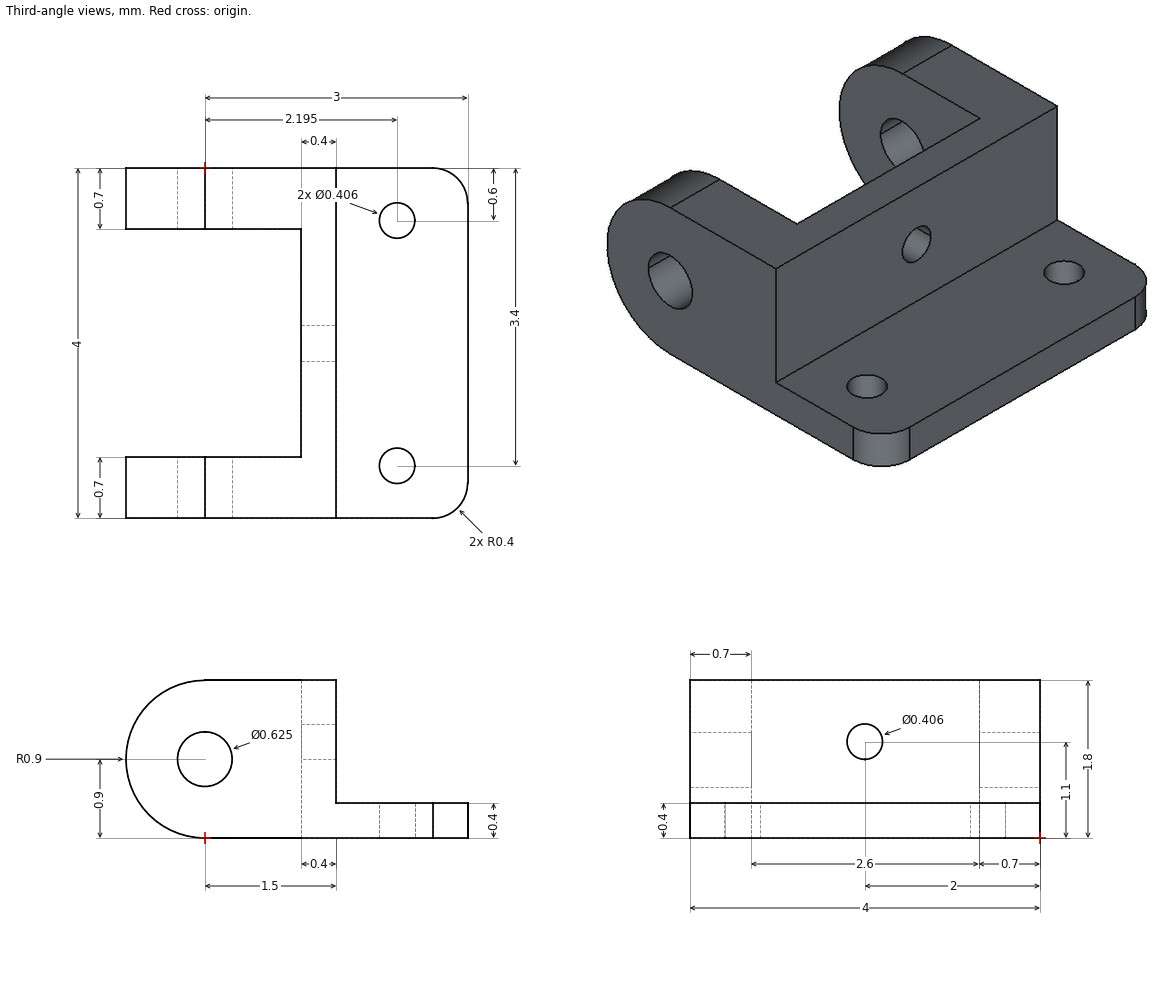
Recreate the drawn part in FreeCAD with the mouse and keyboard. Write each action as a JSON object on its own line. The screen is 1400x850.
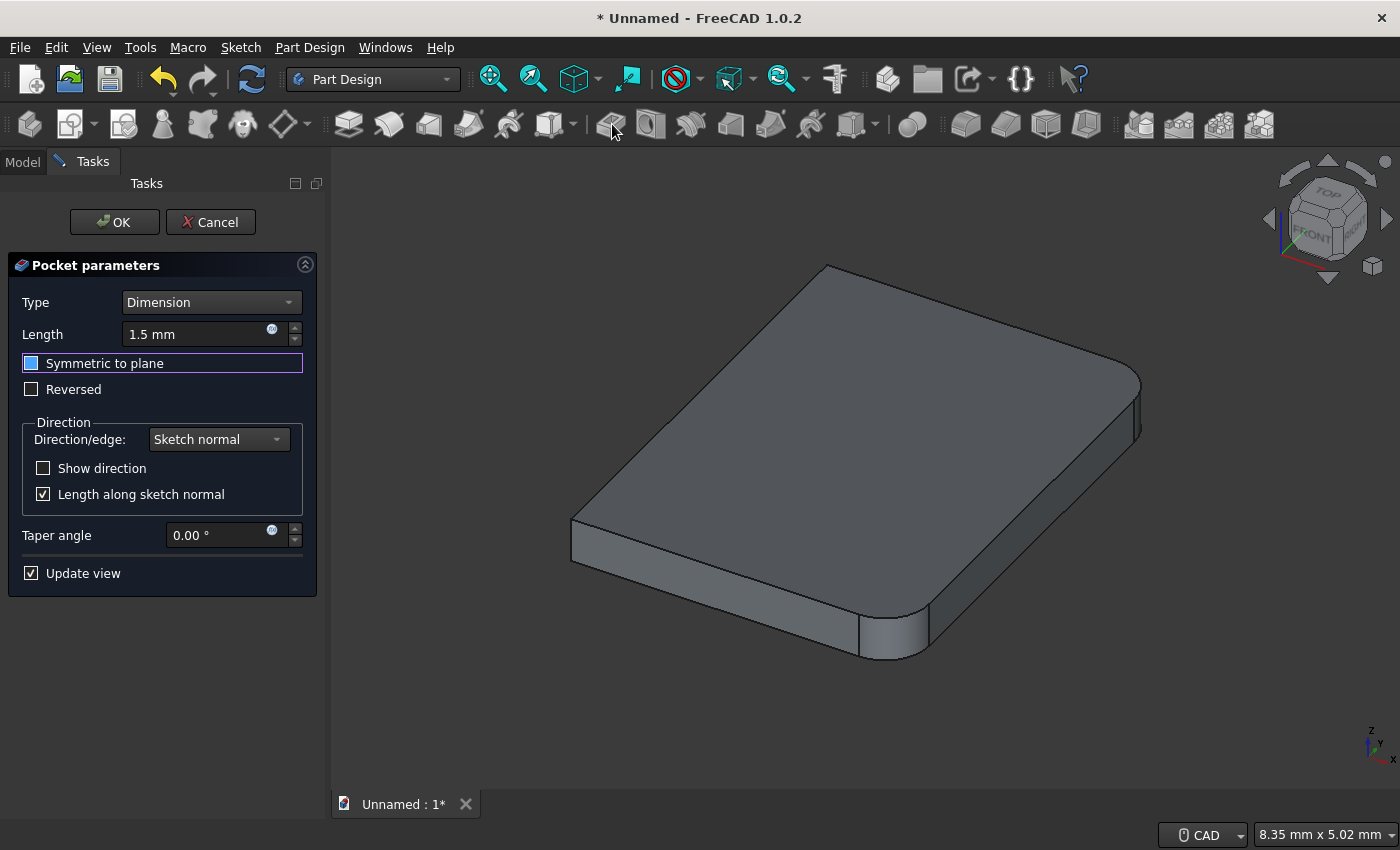
{"action": "left_click", "coordinate": [30, 389]}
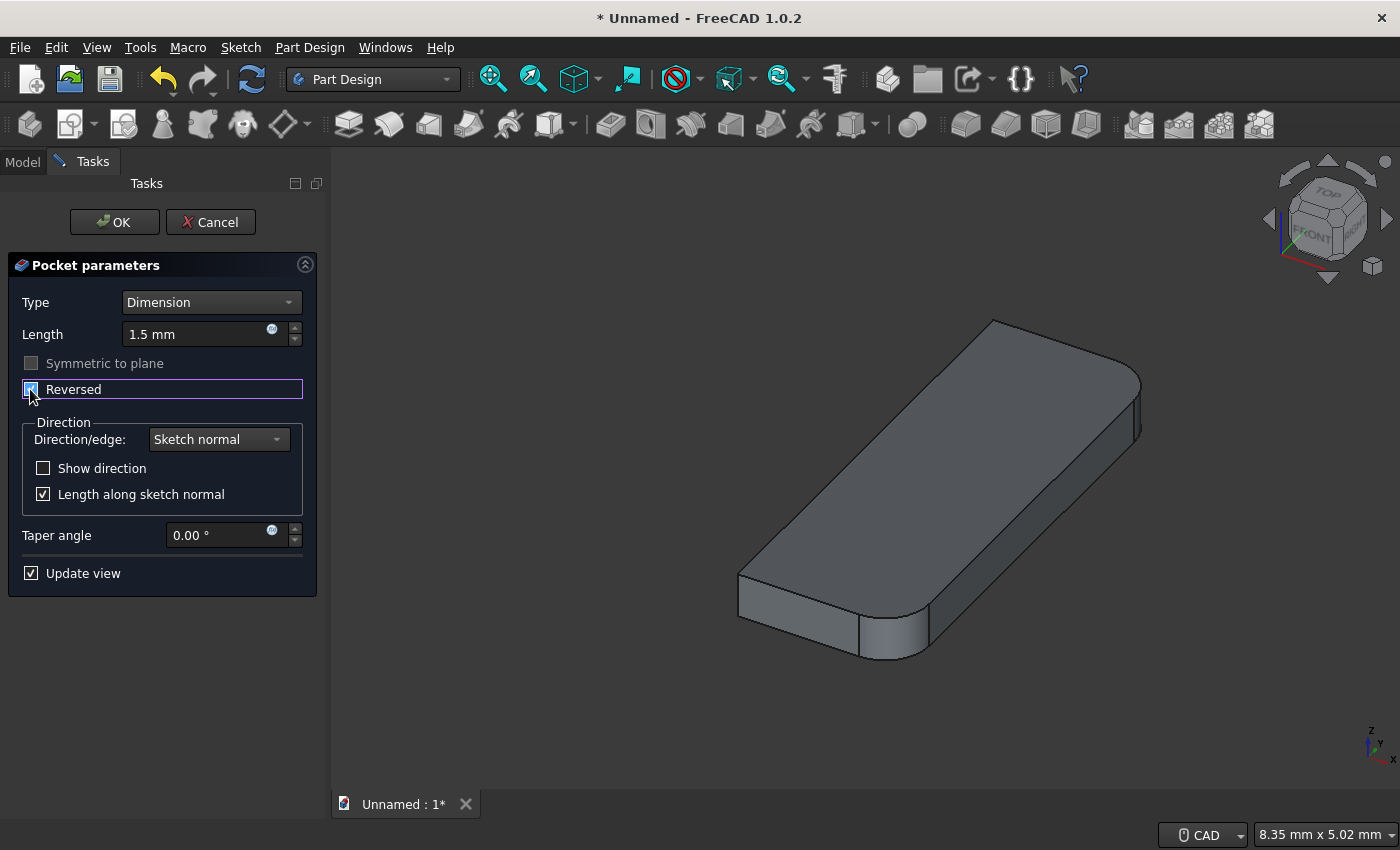
{"action": "left_click", "coordinate": [115, 222]}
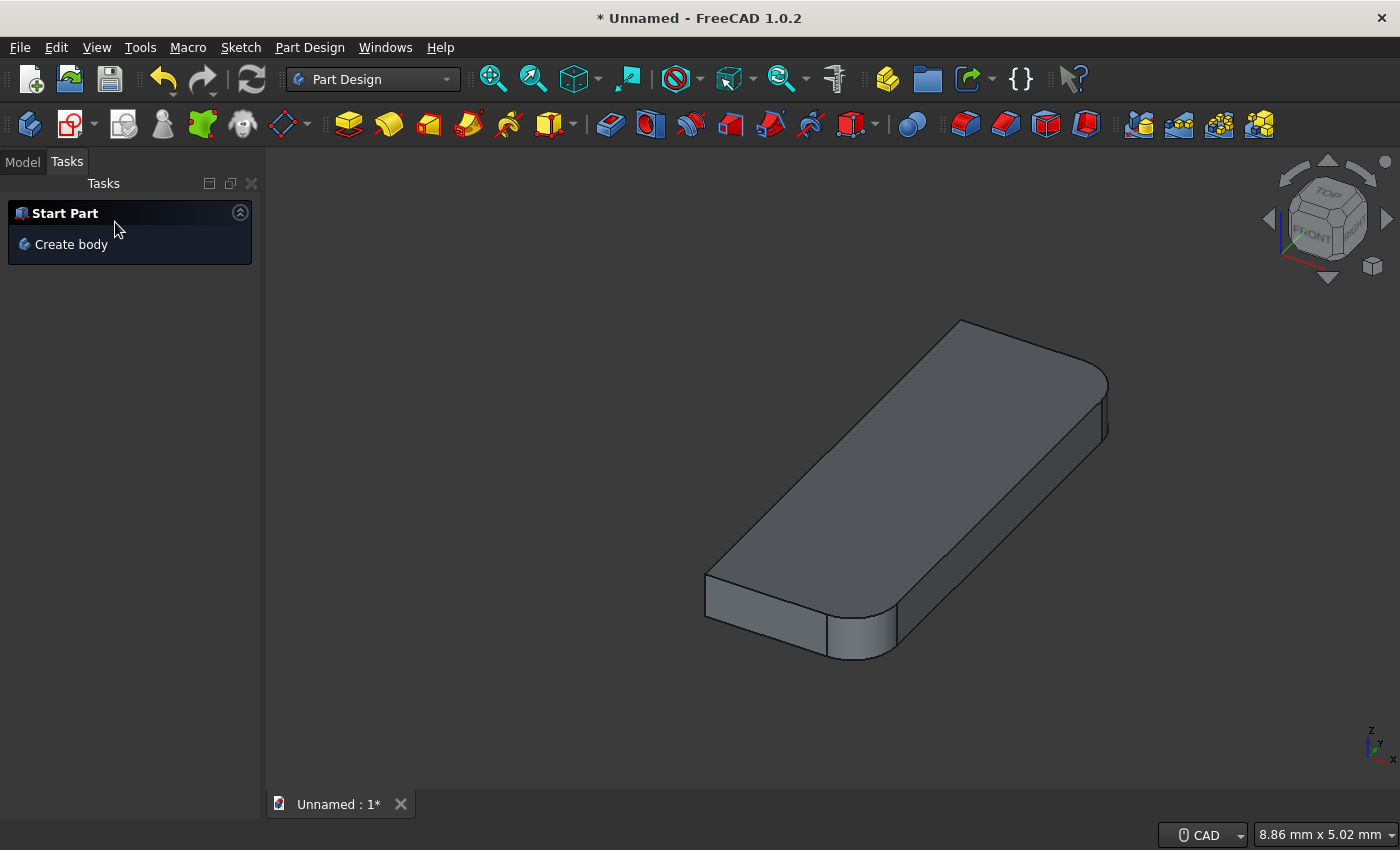
{"action": "left_click", "coordinate": [70, 124]}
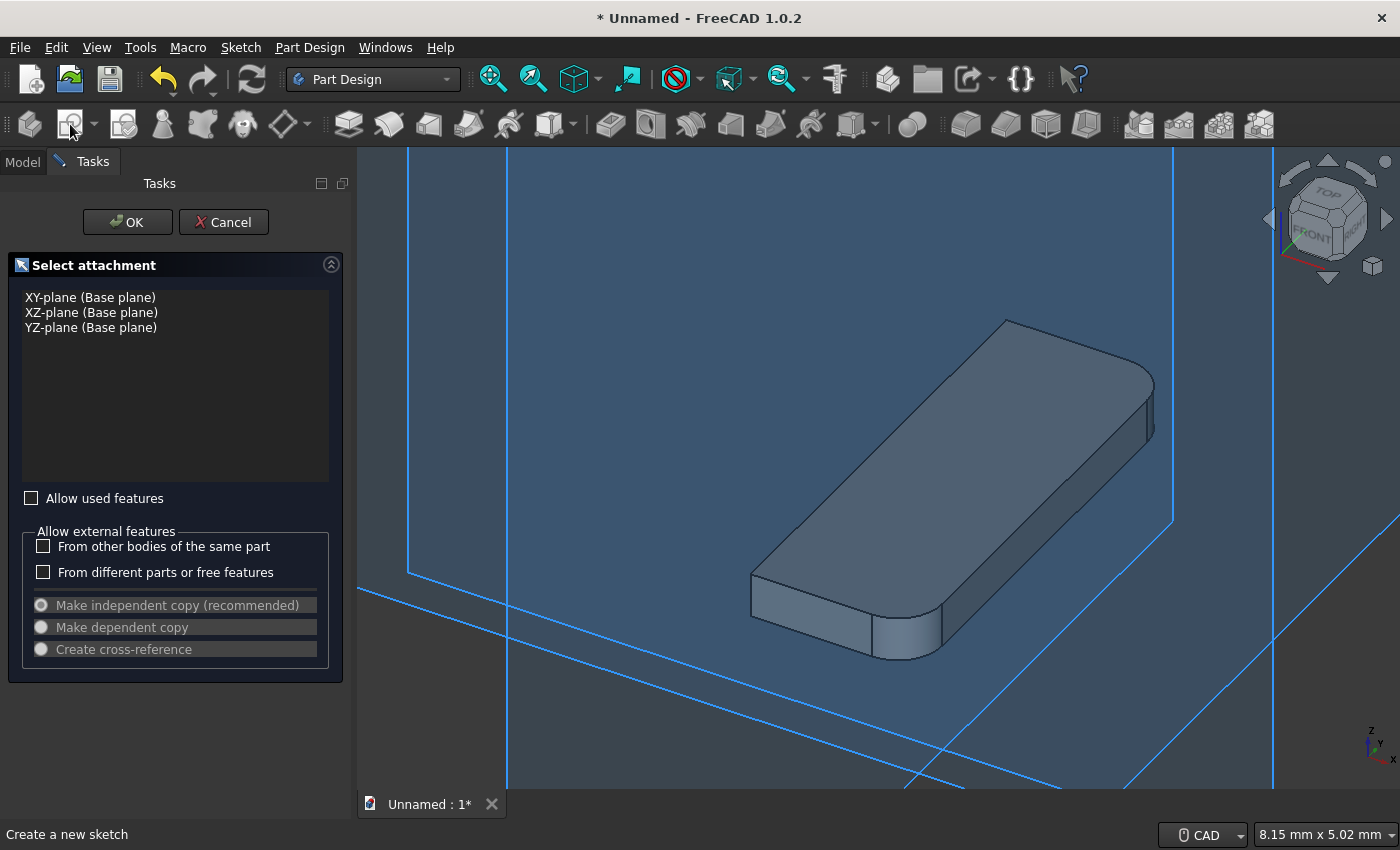
{"action": "left_click", "coordinate": [82, 312]}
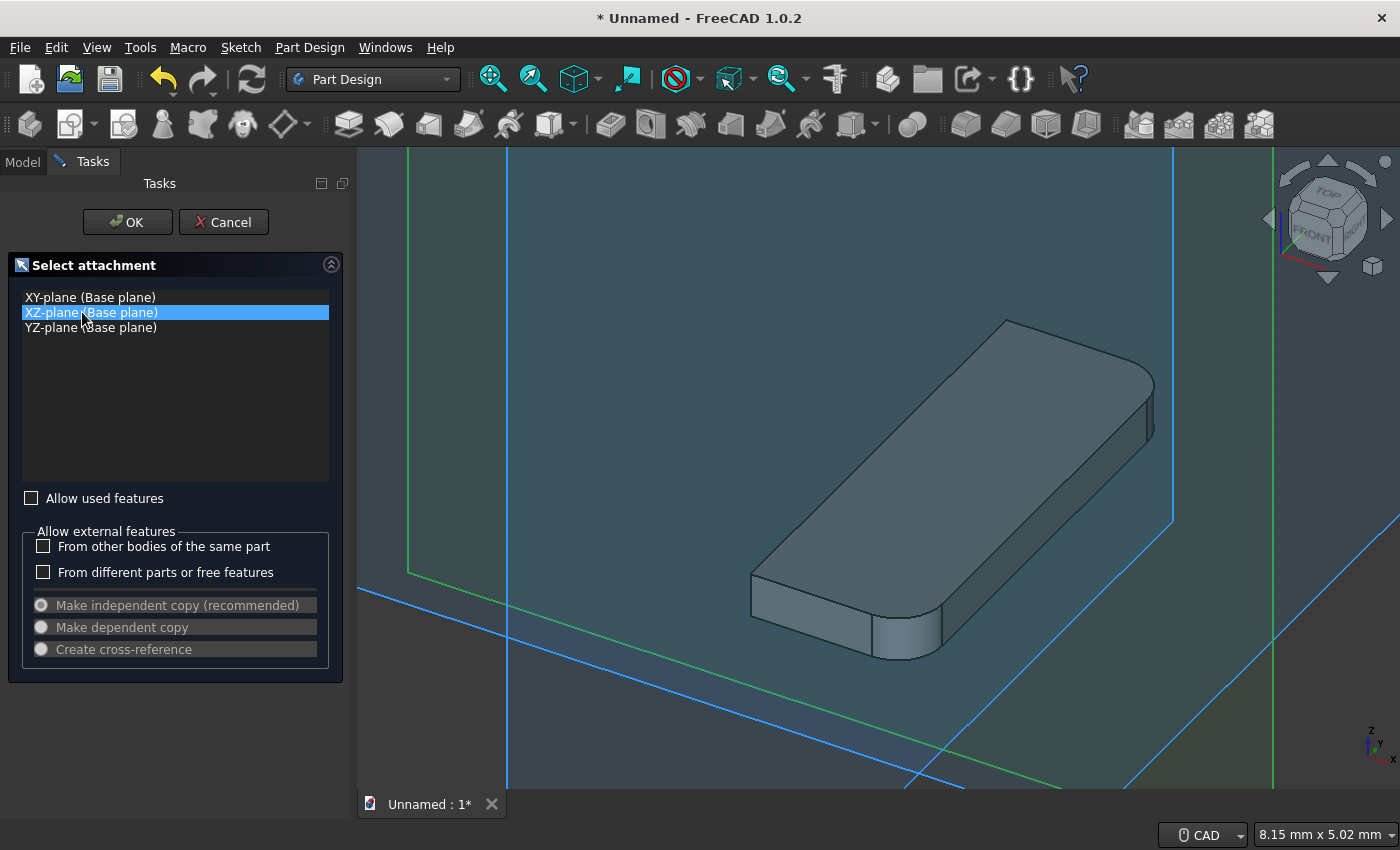
{"action": "left_click", "coordinate": [128, 222]}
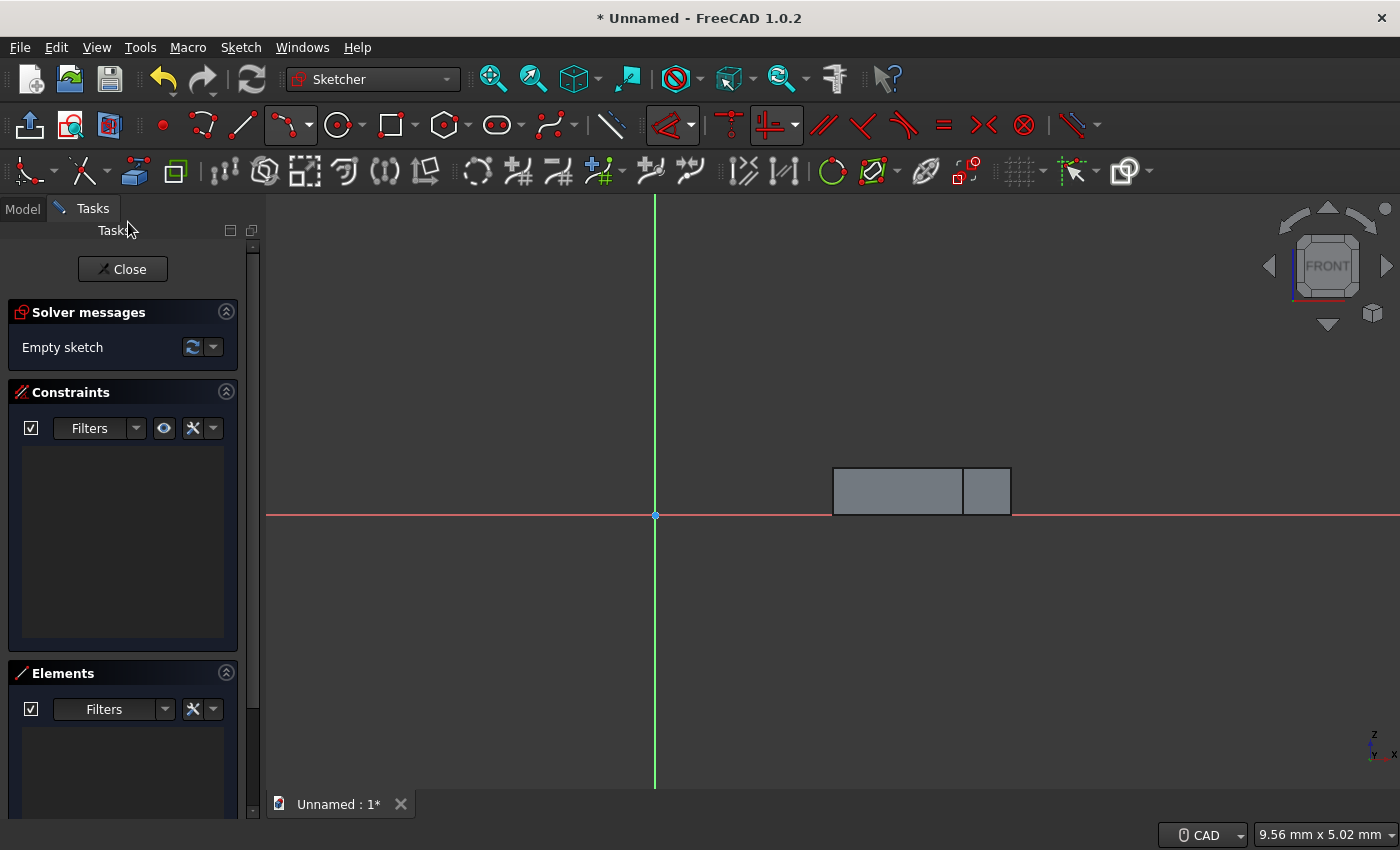
{"action": "key", "text": "q s"}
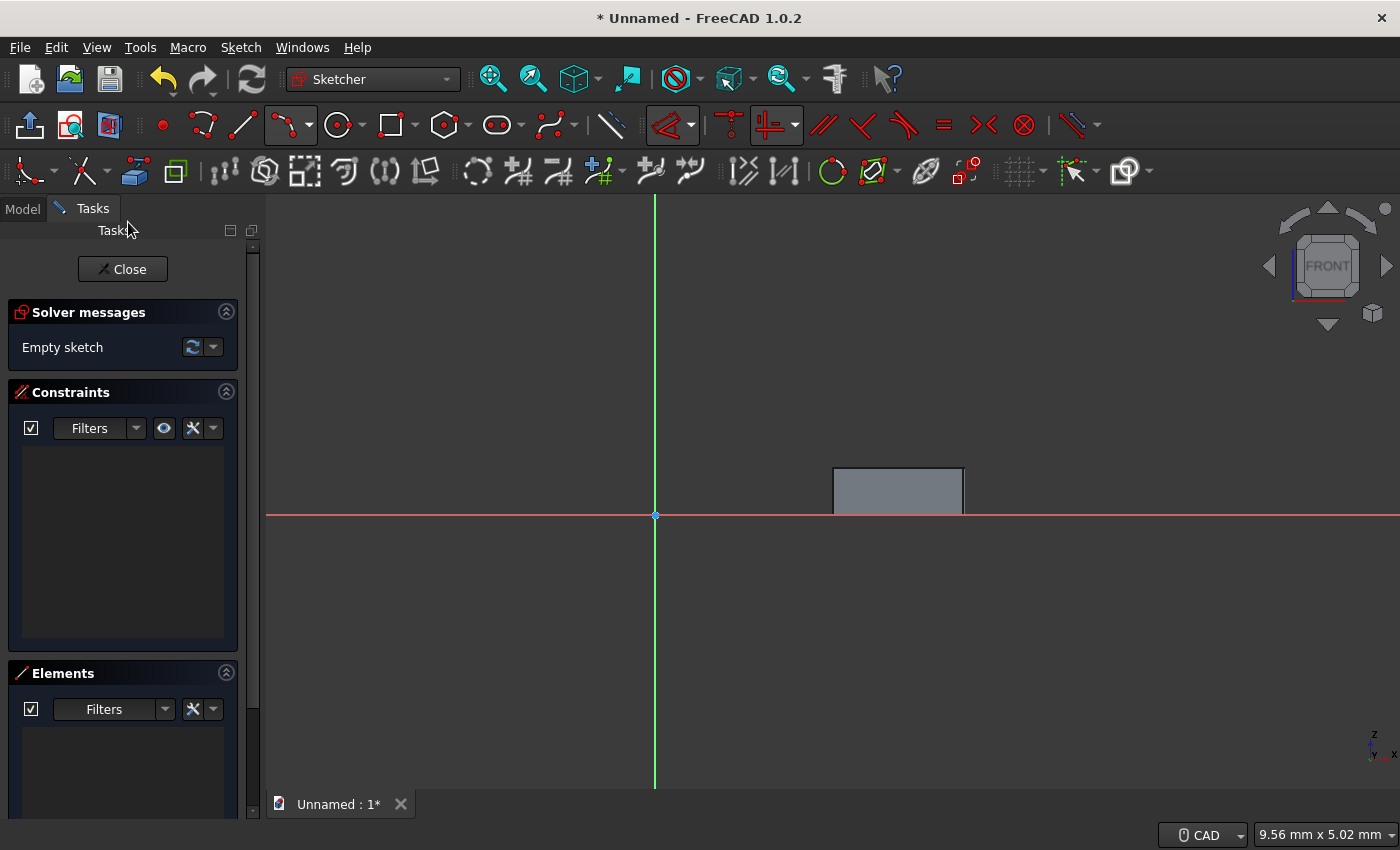
{"action": "scroll", "coordinate": [601, 307], "scroll_direction": "up", "scroll_amount": 3}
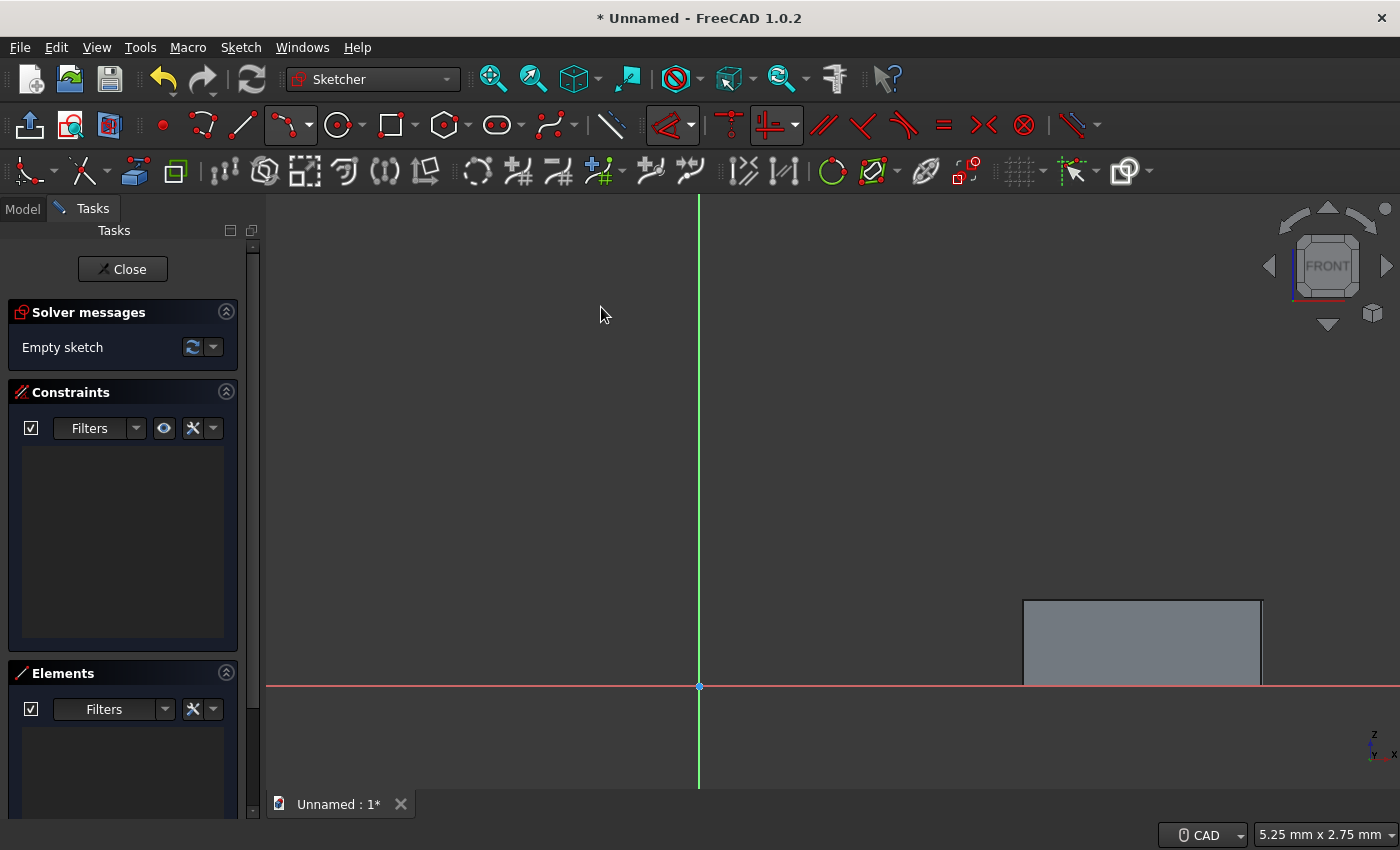
{"action": "key", "text": "g m"}